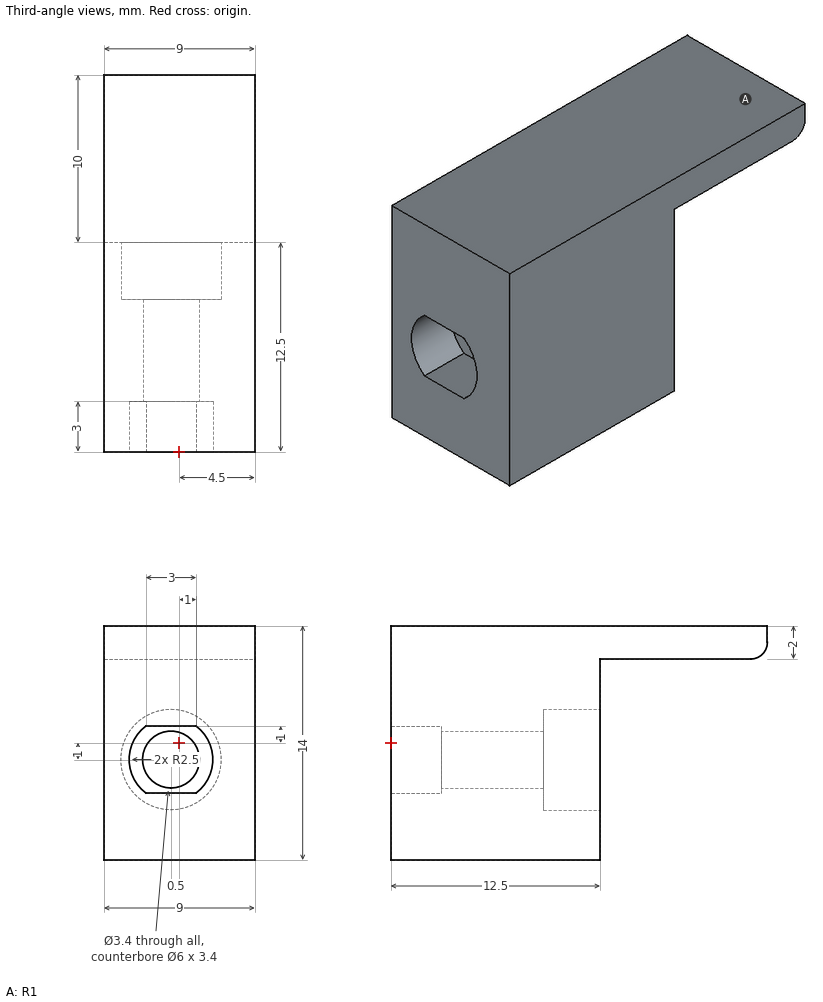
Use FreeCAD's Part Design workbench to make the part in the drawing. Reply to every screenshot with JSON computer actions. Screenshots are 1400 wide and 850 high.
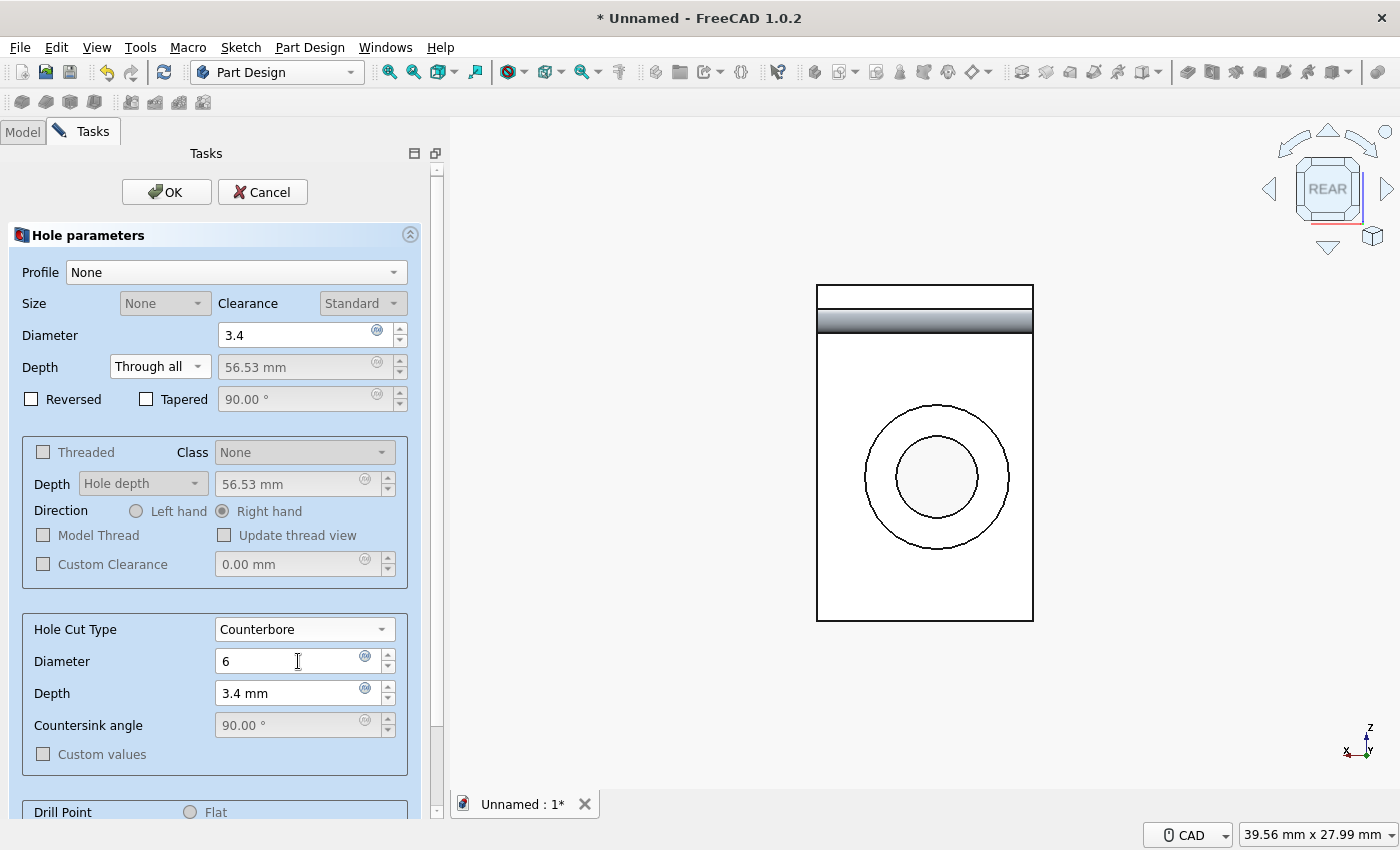
{"action": "left_click", "coordinate": [167, 192]}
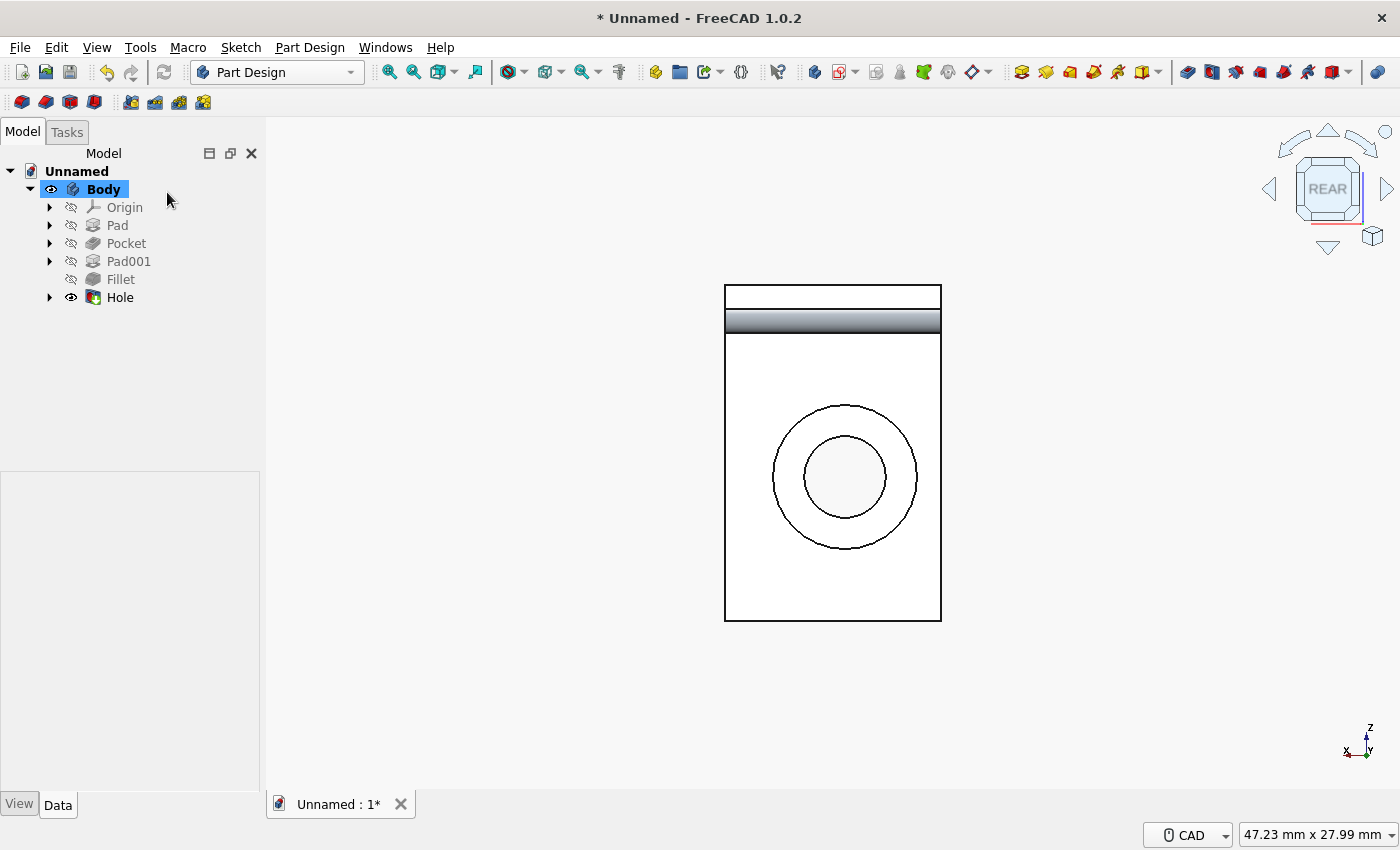
{"action": "key", "text": "0"}